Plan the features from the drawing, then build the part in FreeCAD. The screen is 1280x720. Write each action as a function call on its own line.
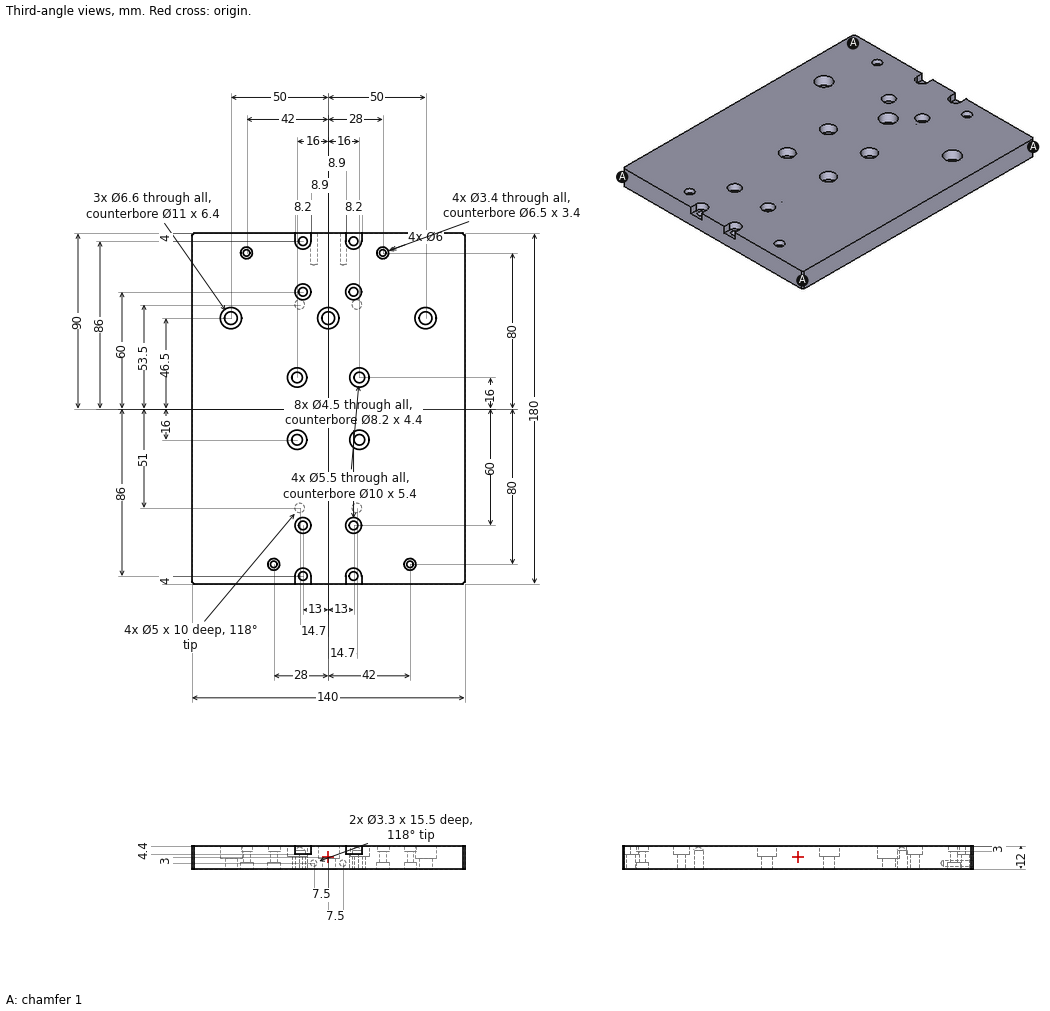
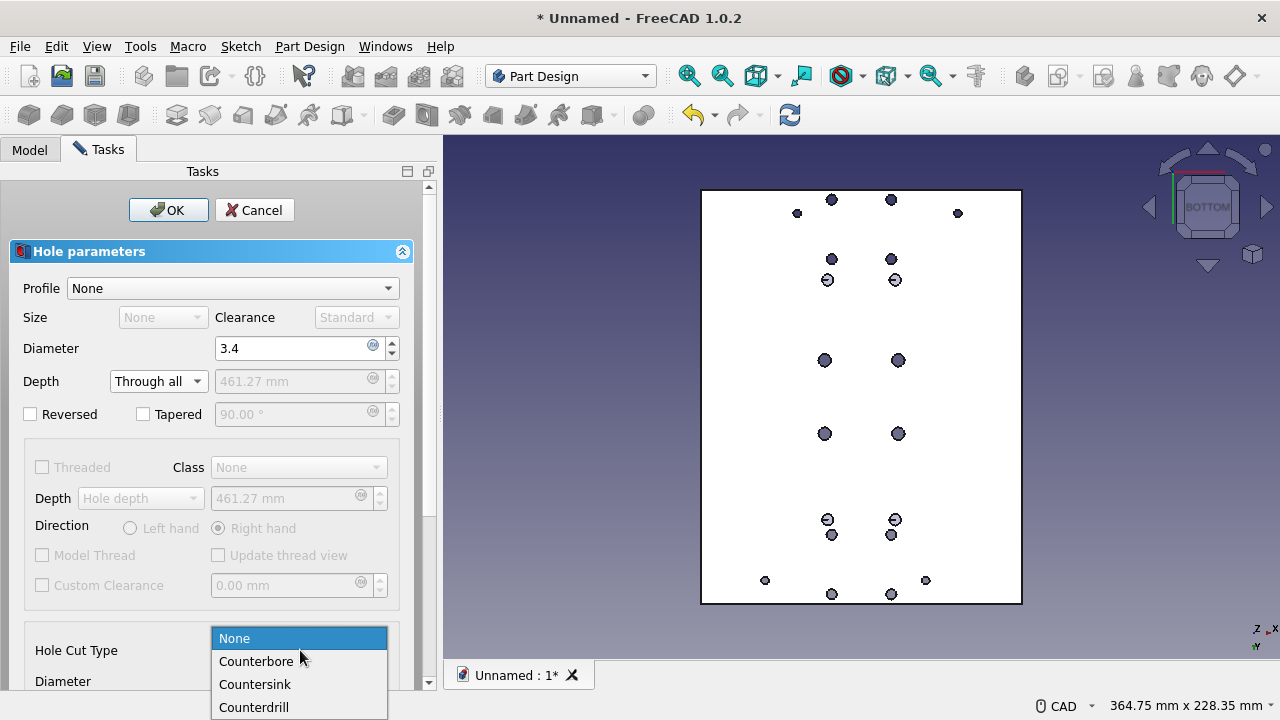
click(298, 662)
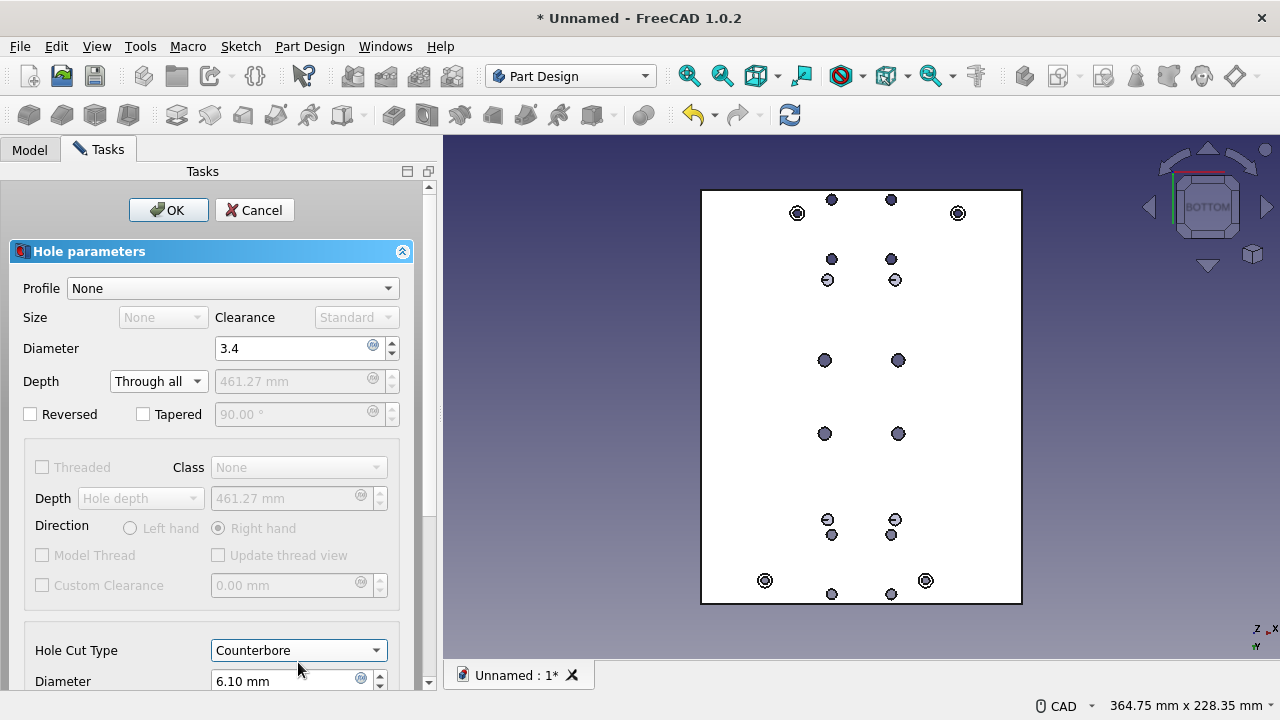
scroll(429, 436, down, 2)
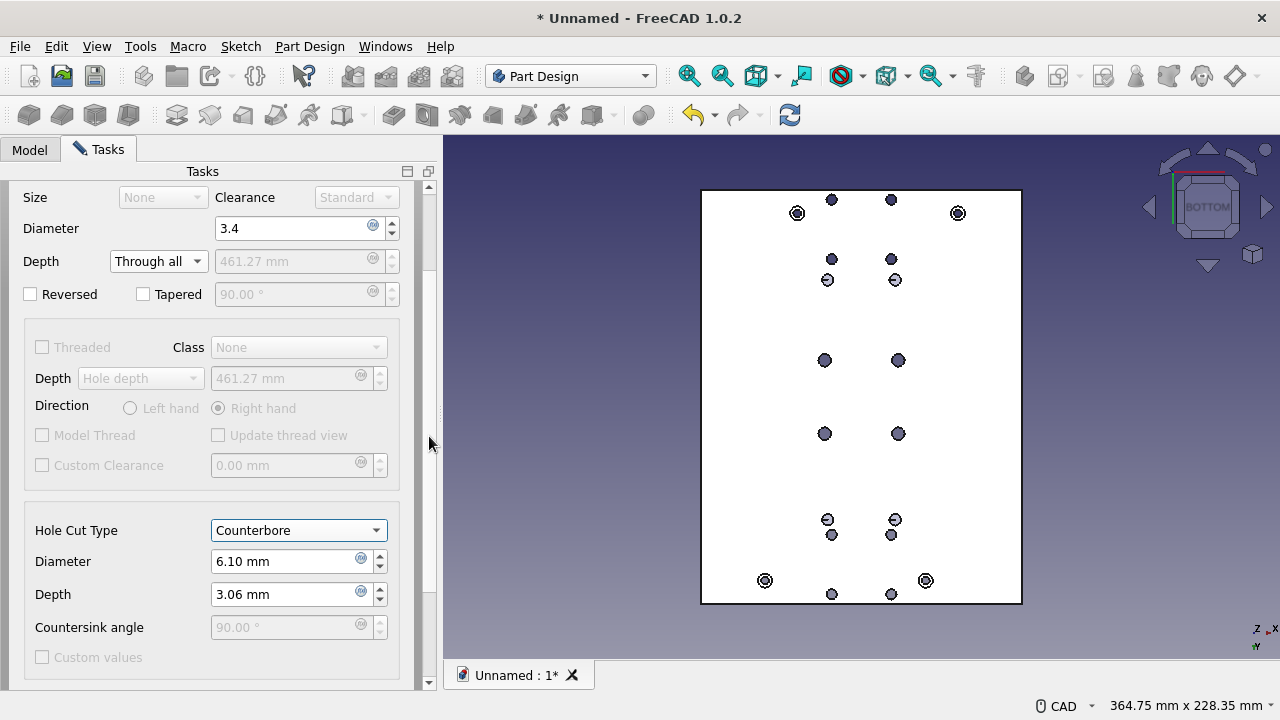
triple_click(292, 562)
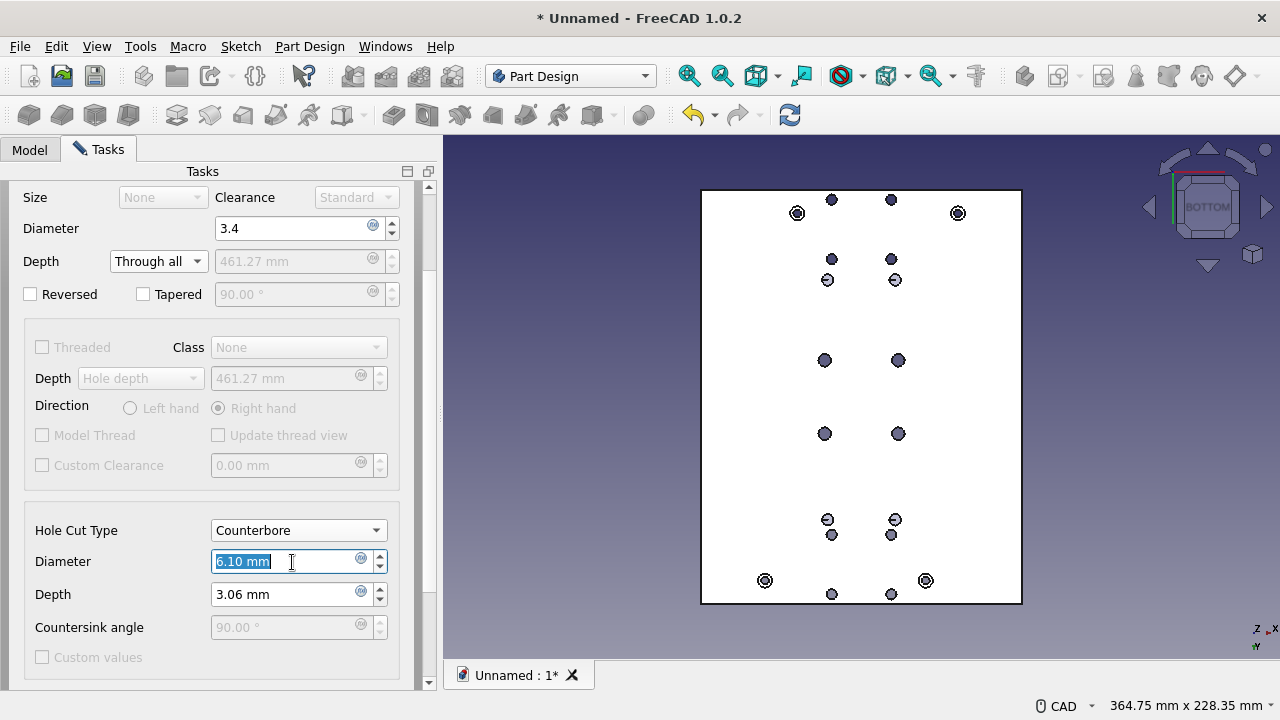
text(6.5)
key(Tab)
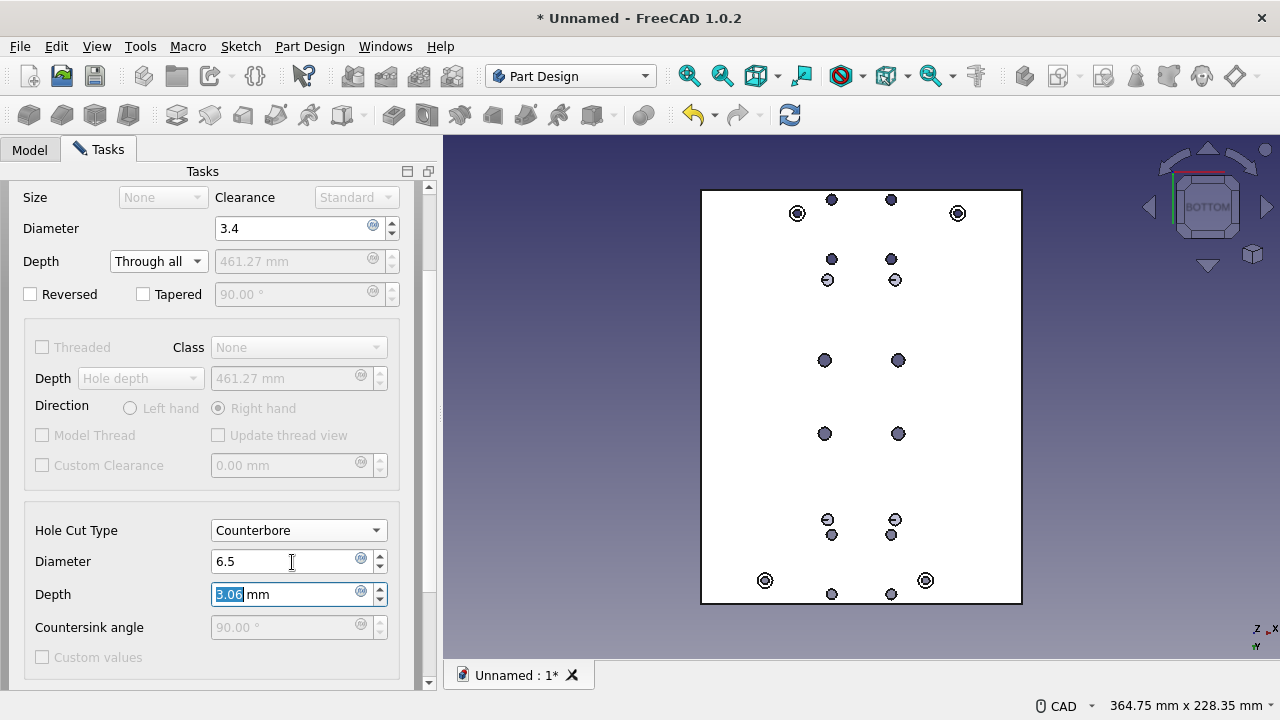
text(3.4)
key(Tab)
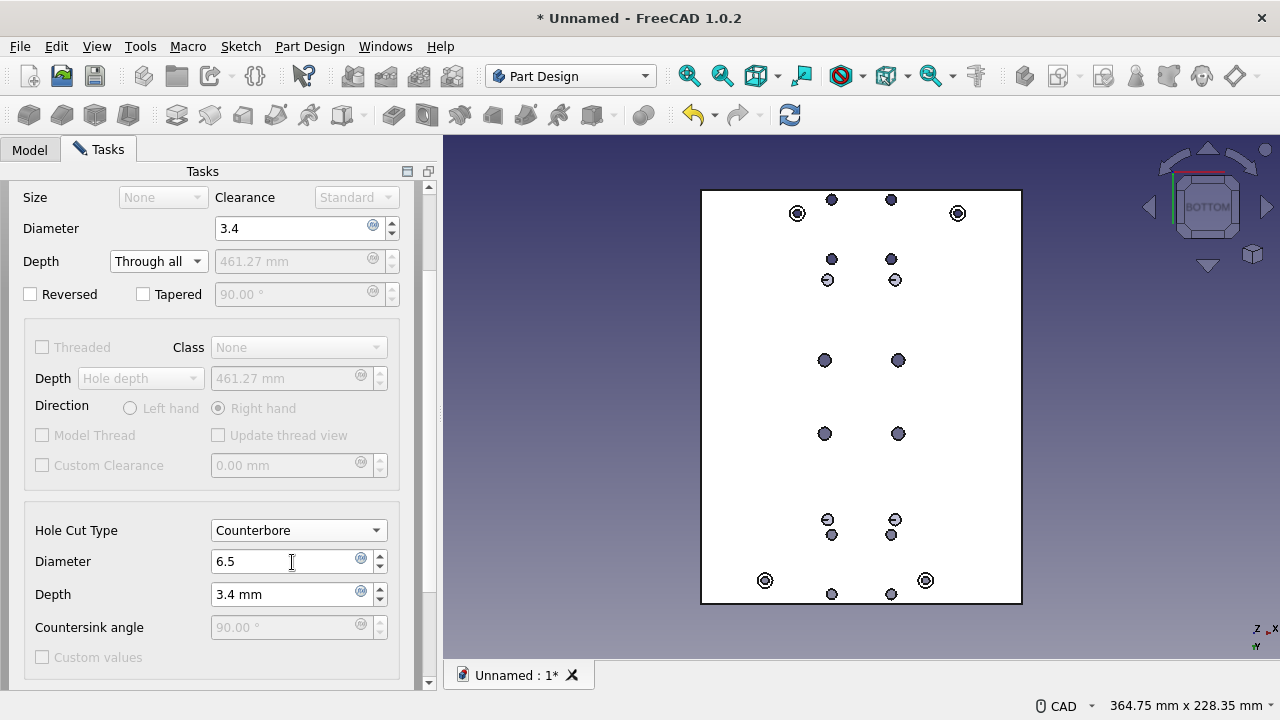
scroll(429, 436, up, 3)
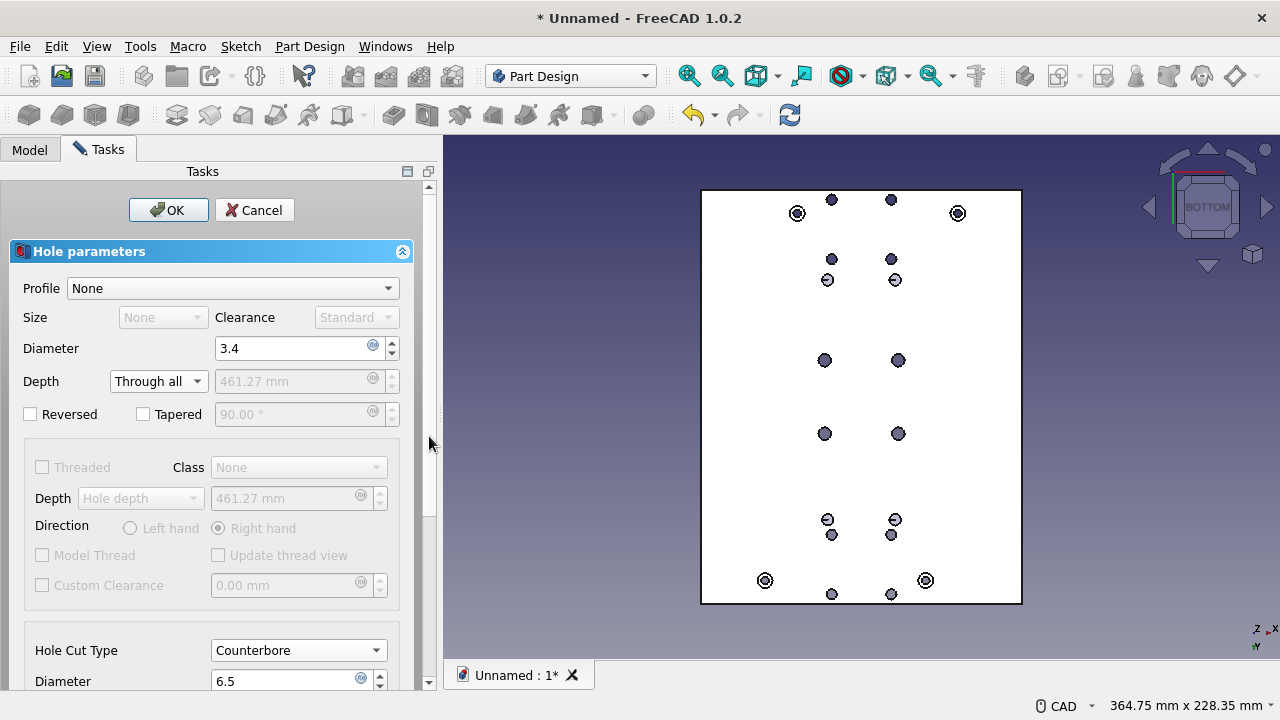
click(169, 210)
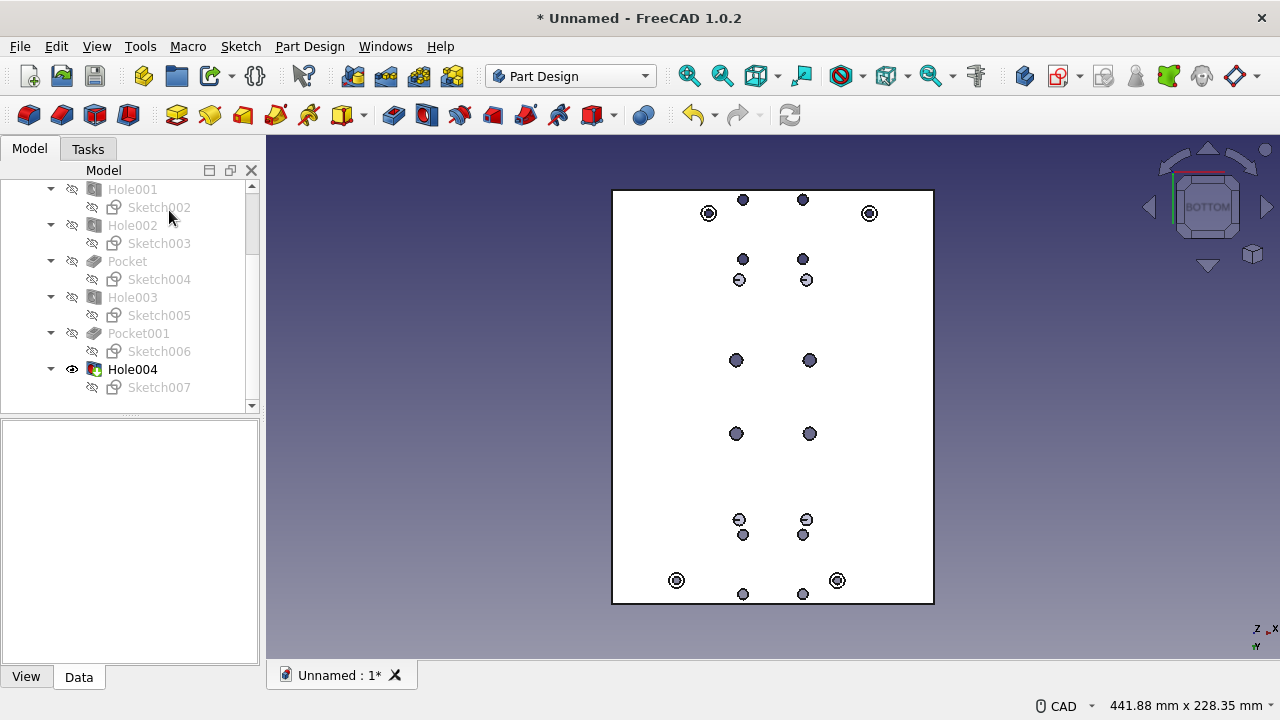
key(0)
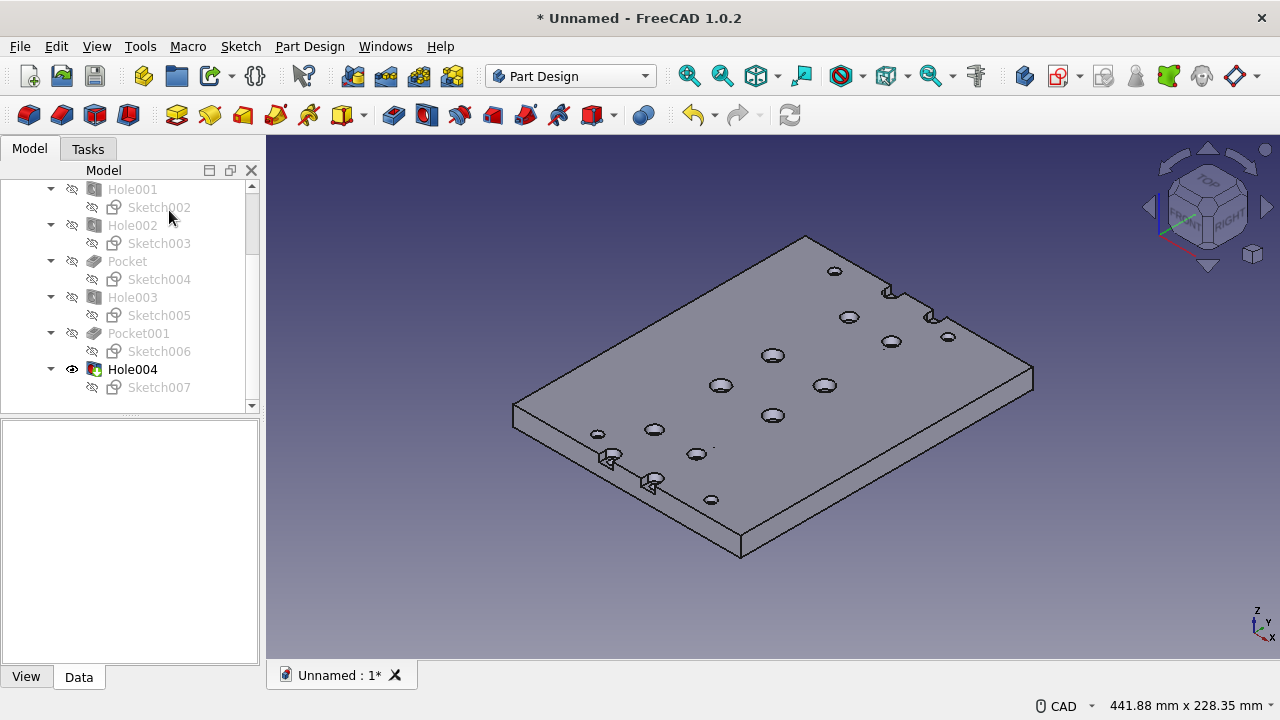
click(741, 546)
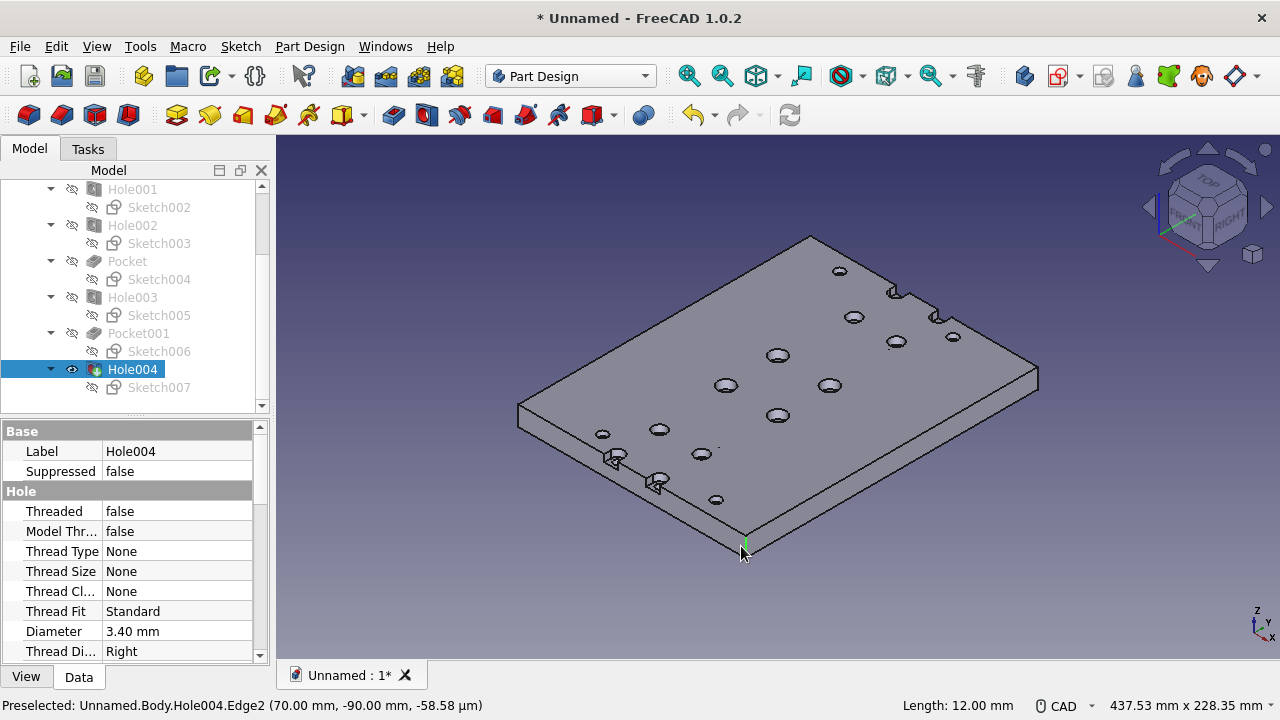
key(2)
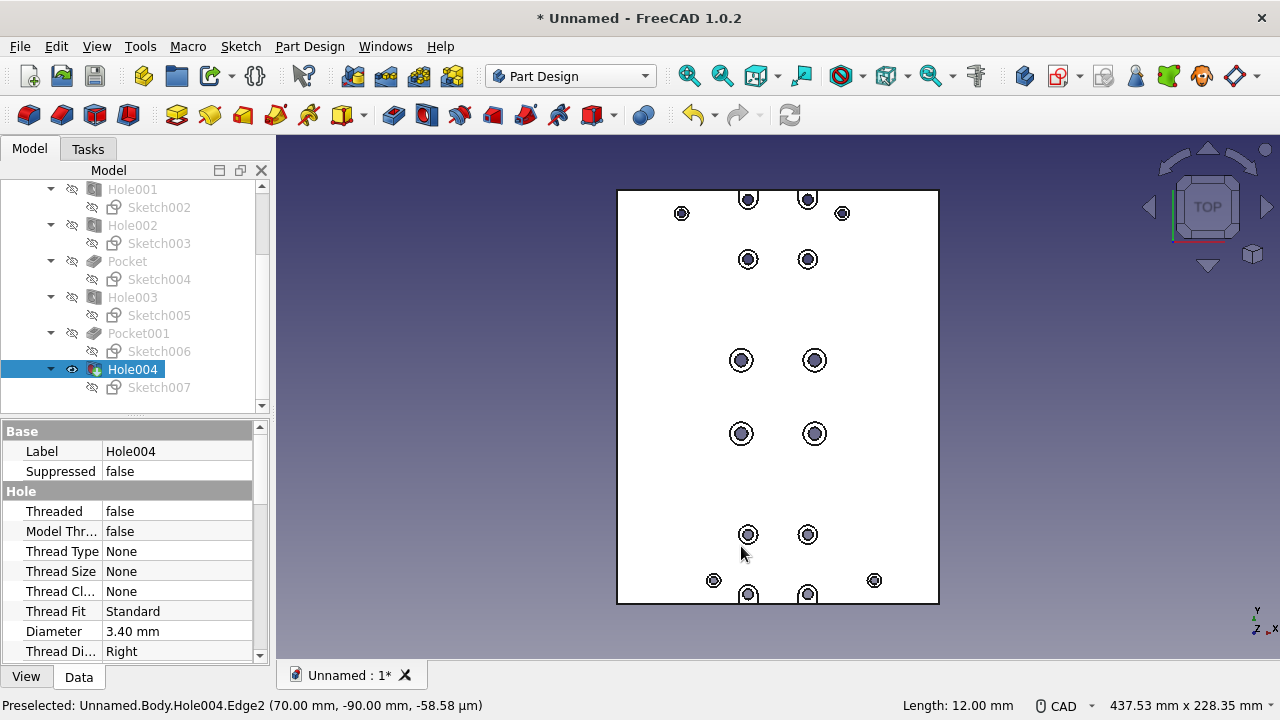
key(1)